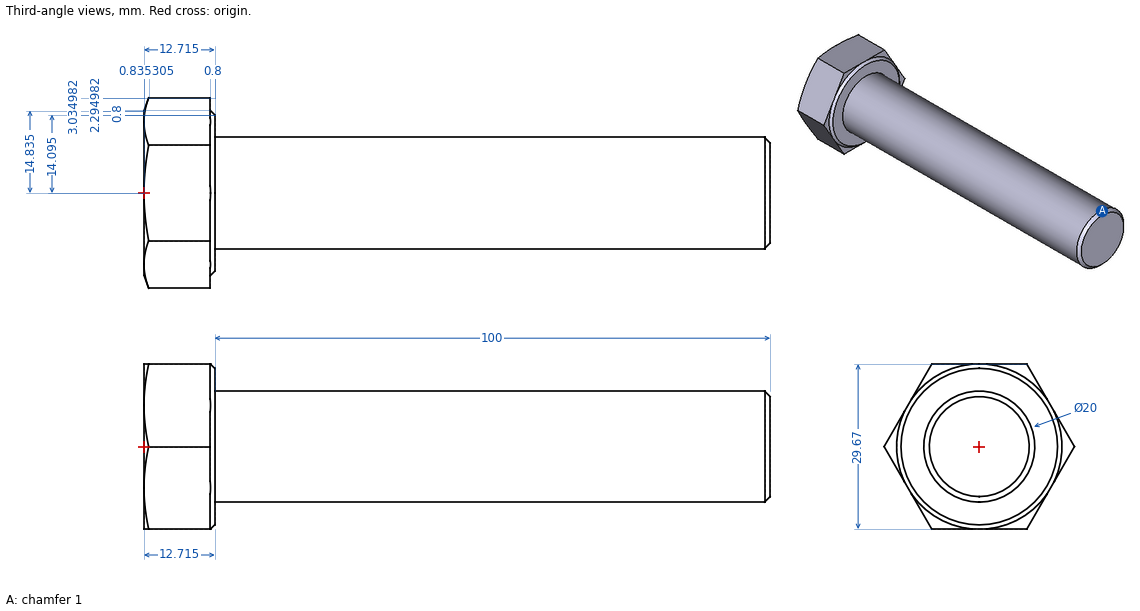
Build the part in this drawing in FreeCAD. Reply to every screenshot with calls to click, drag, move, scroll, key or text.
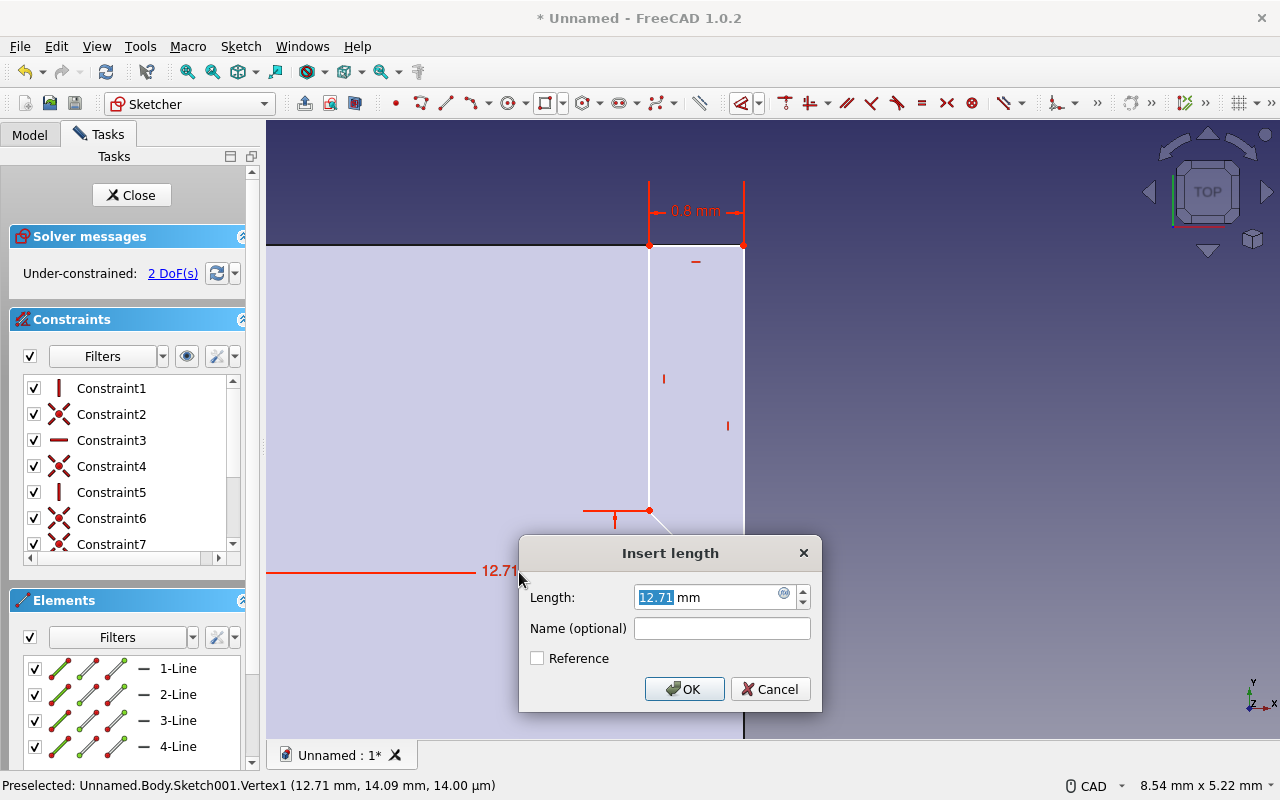
text(12.715)
key(Return)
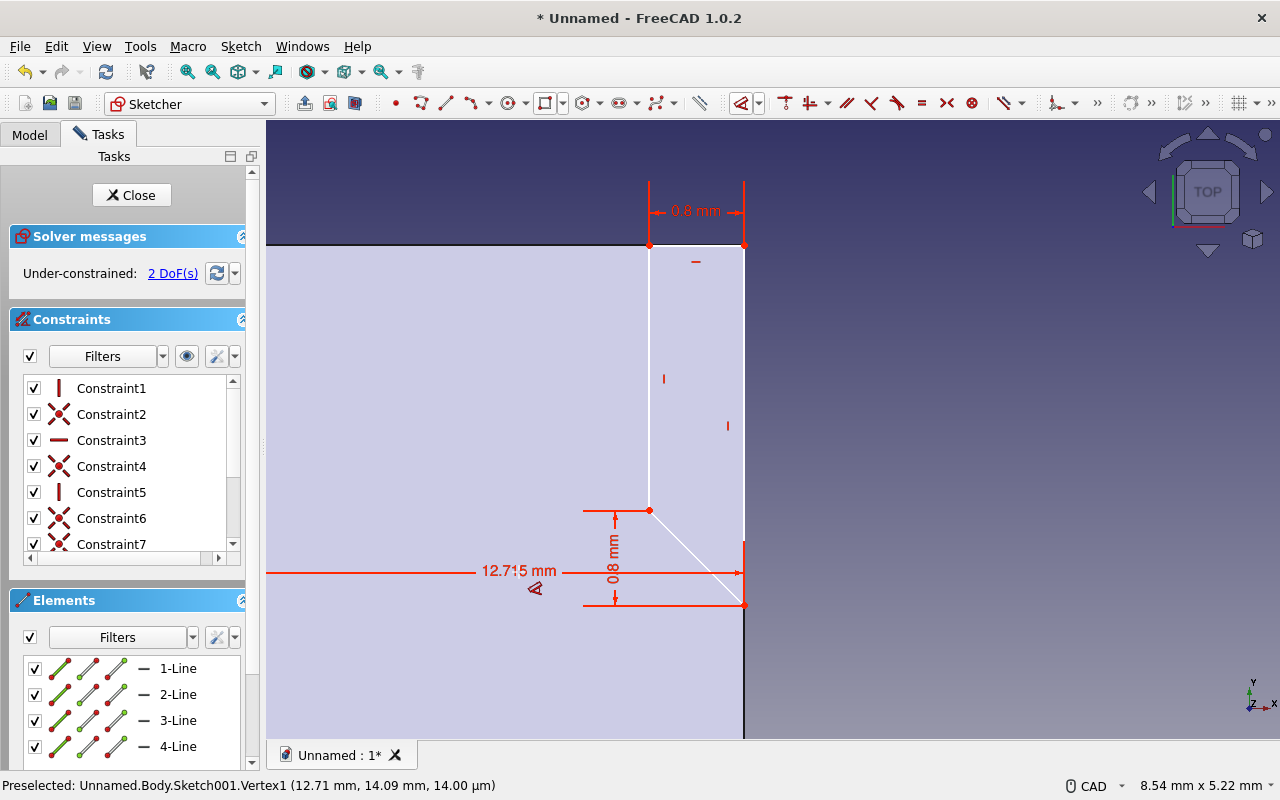
click(744, 606)
click(778, 658)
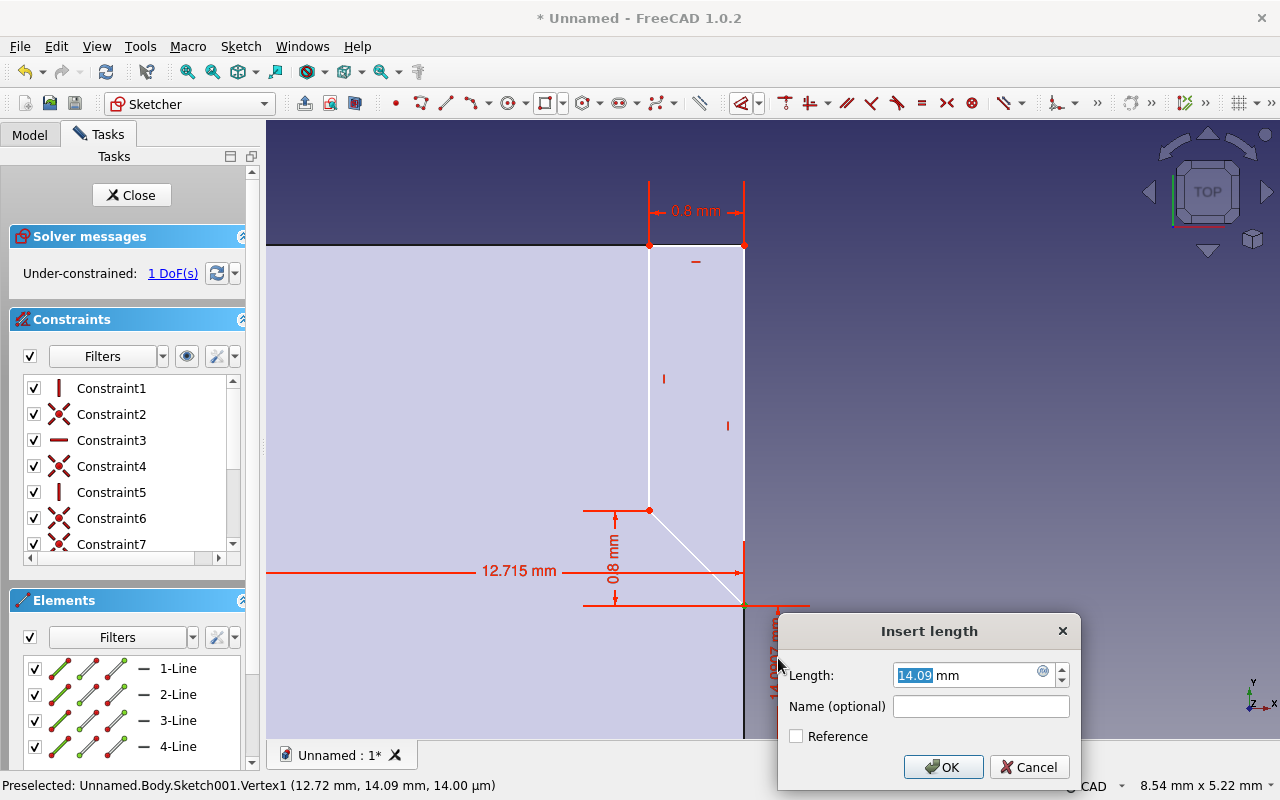
text(14.095)
key(Return)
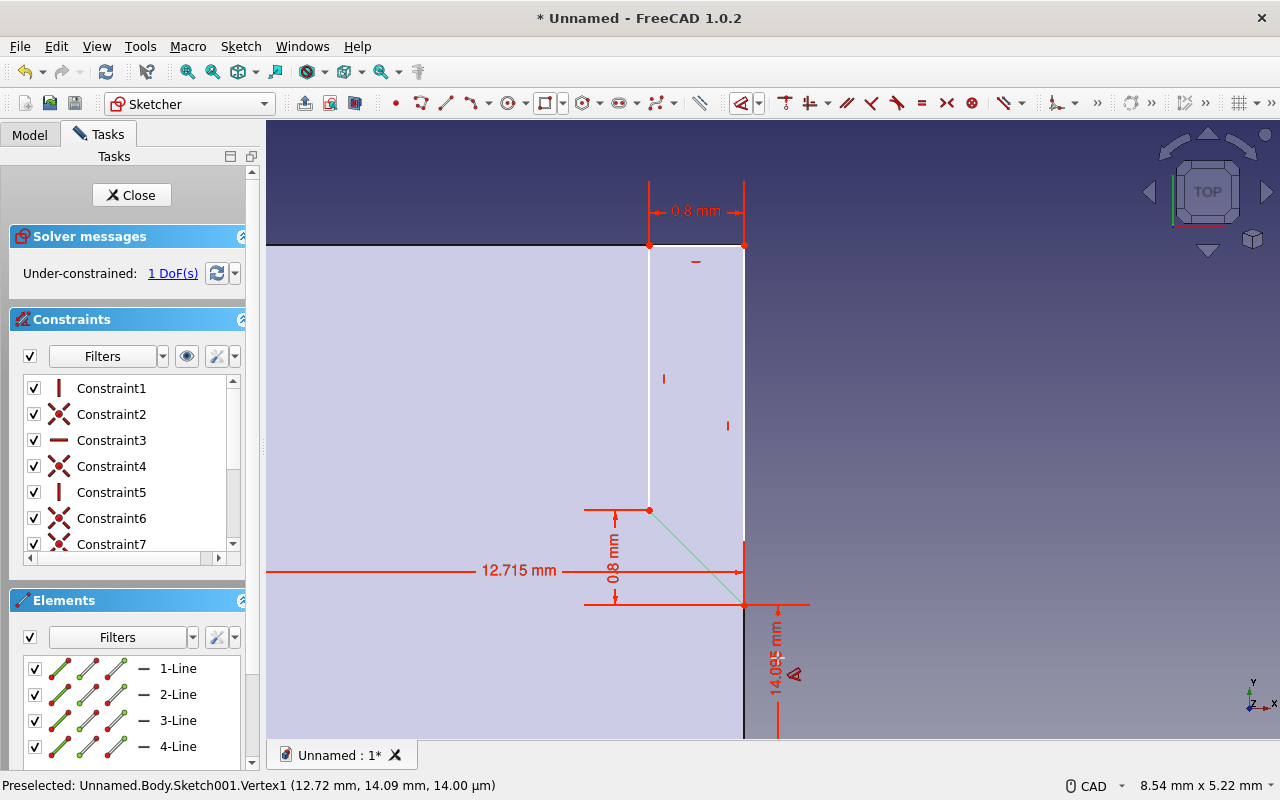
click(744, 498)
click(778, 426)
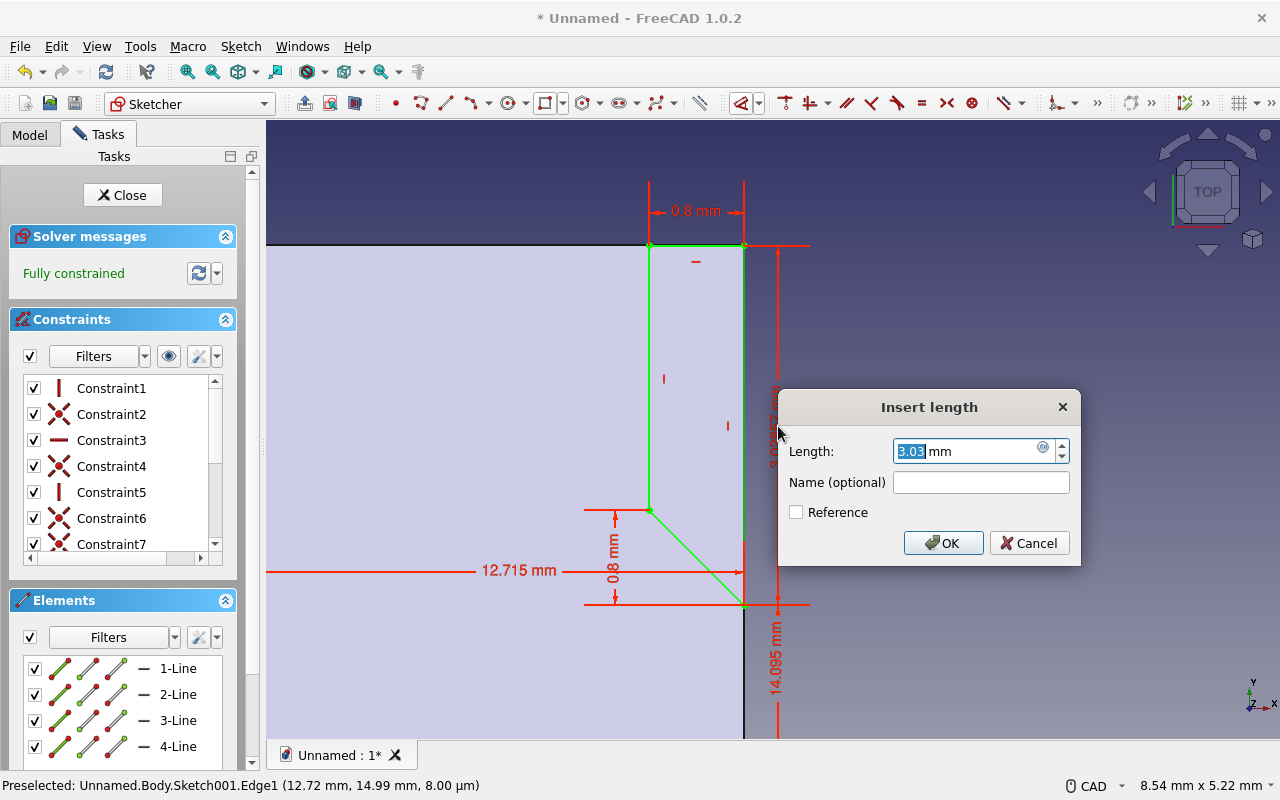
text(3.034982)
key(Return)
key(Escape)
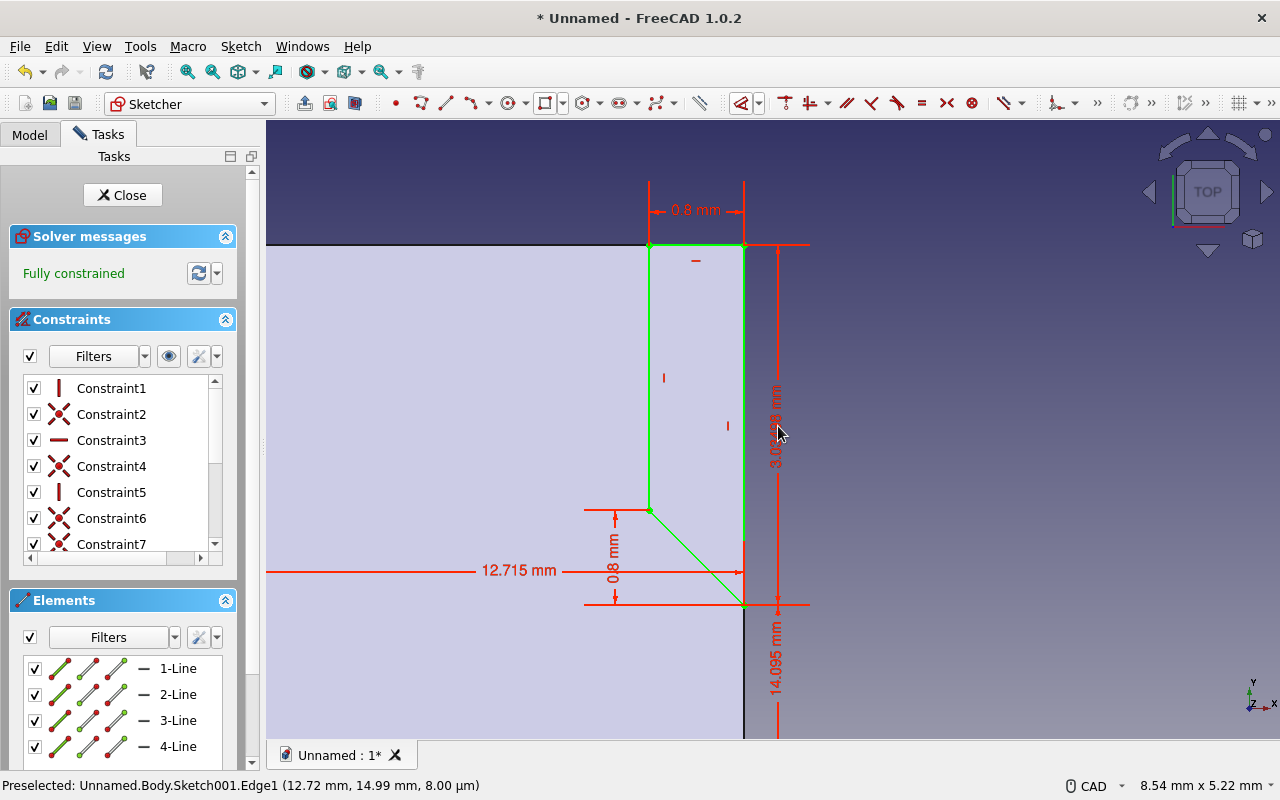
click(123, 195)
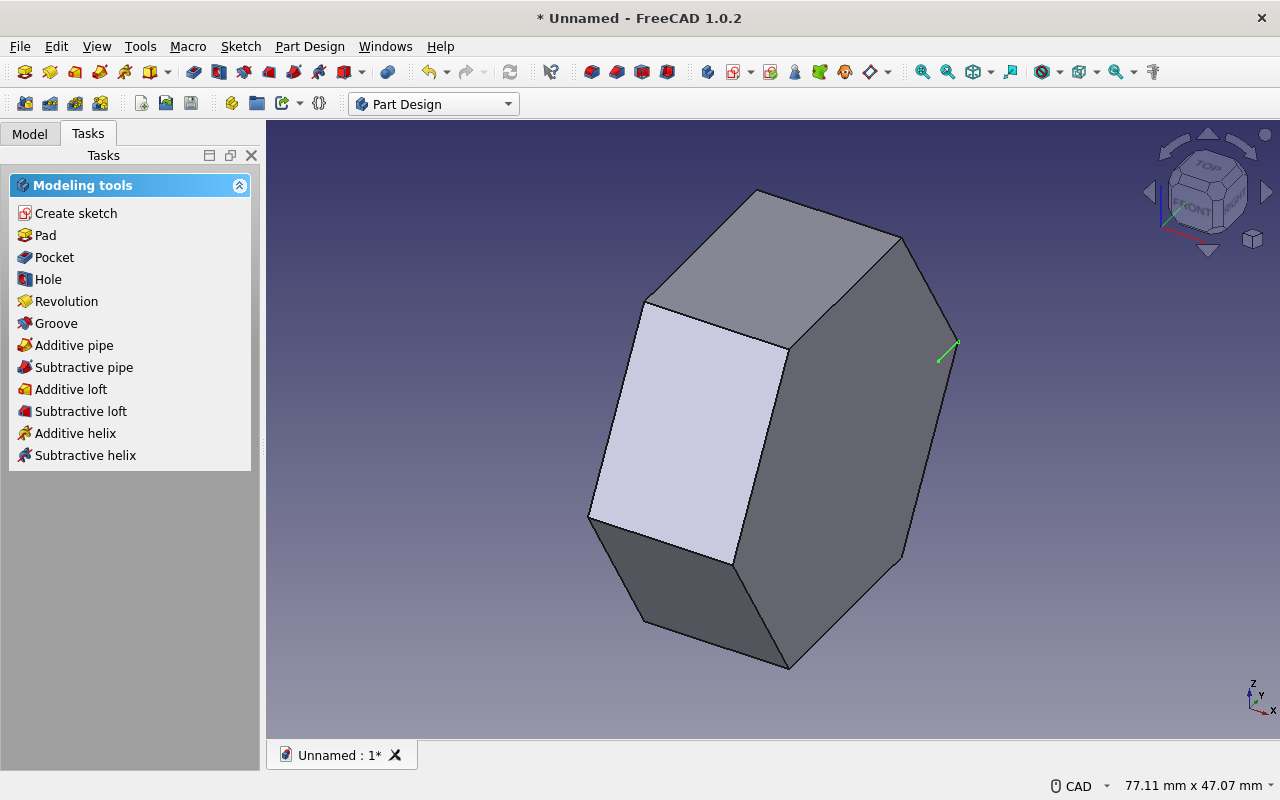
click(244, 72)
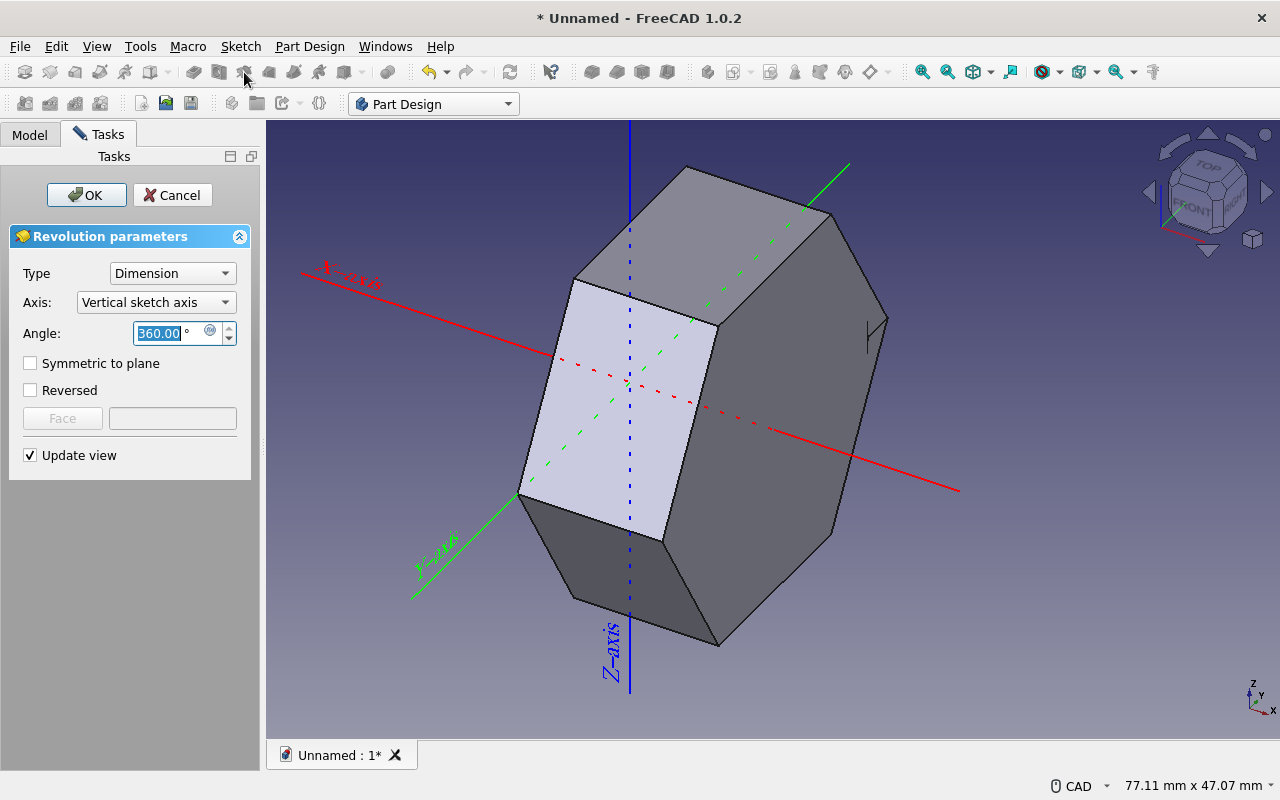
click(157, 302)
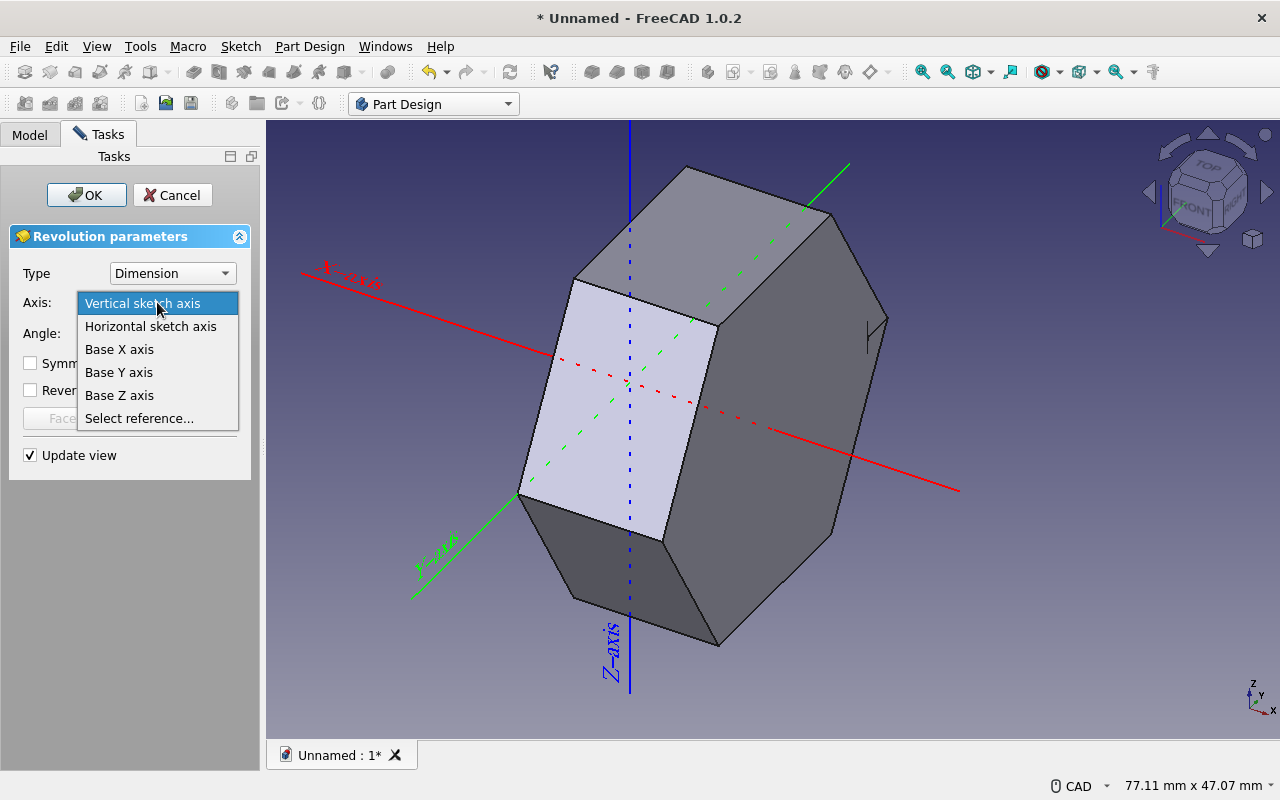
click(156, 326)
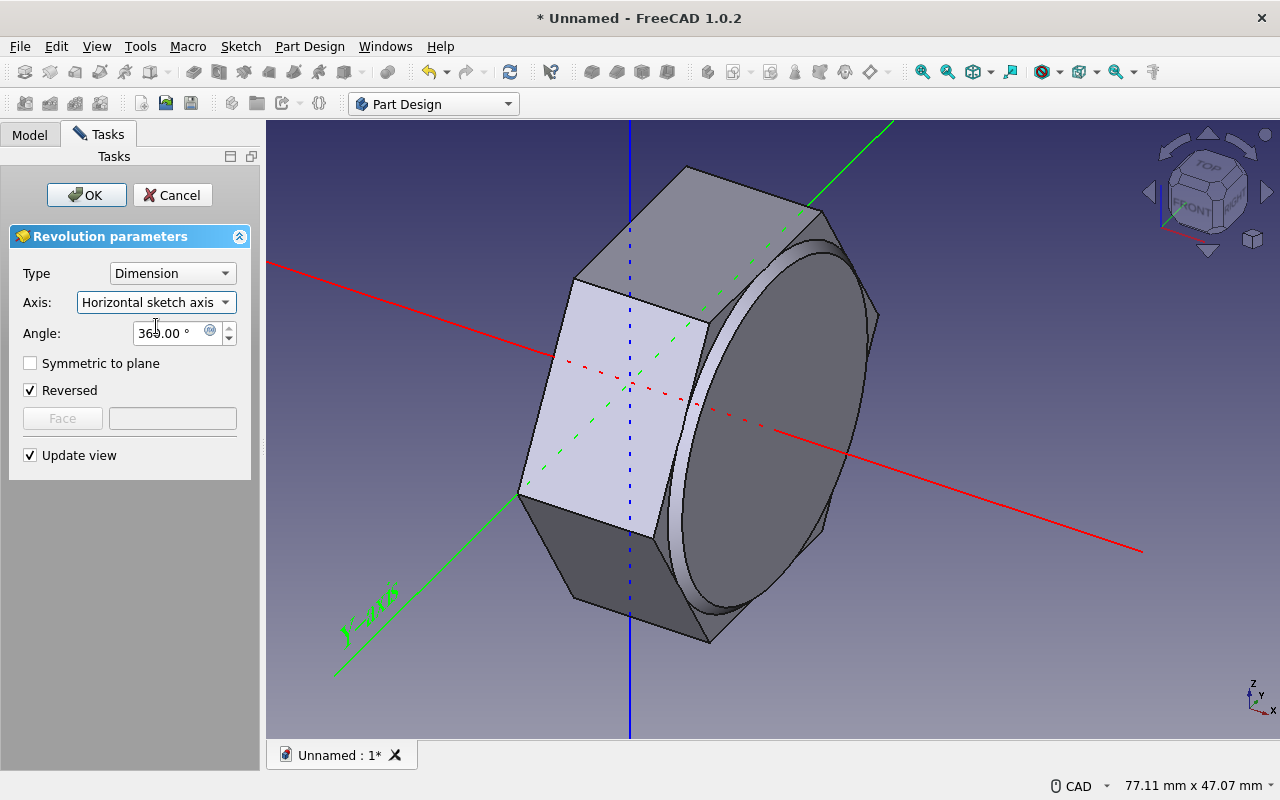
click(87, 195)